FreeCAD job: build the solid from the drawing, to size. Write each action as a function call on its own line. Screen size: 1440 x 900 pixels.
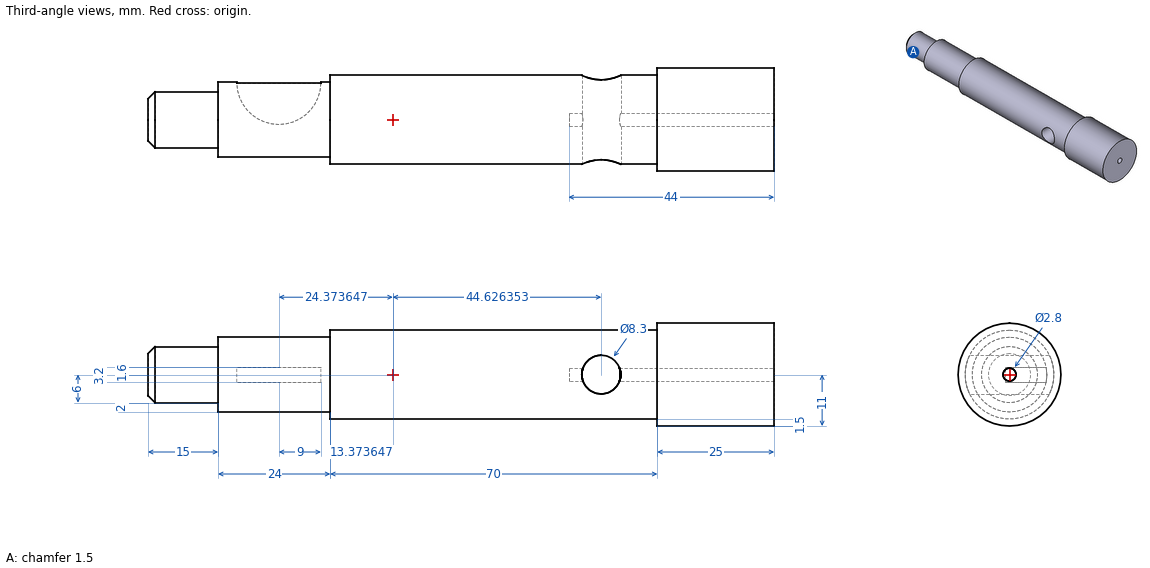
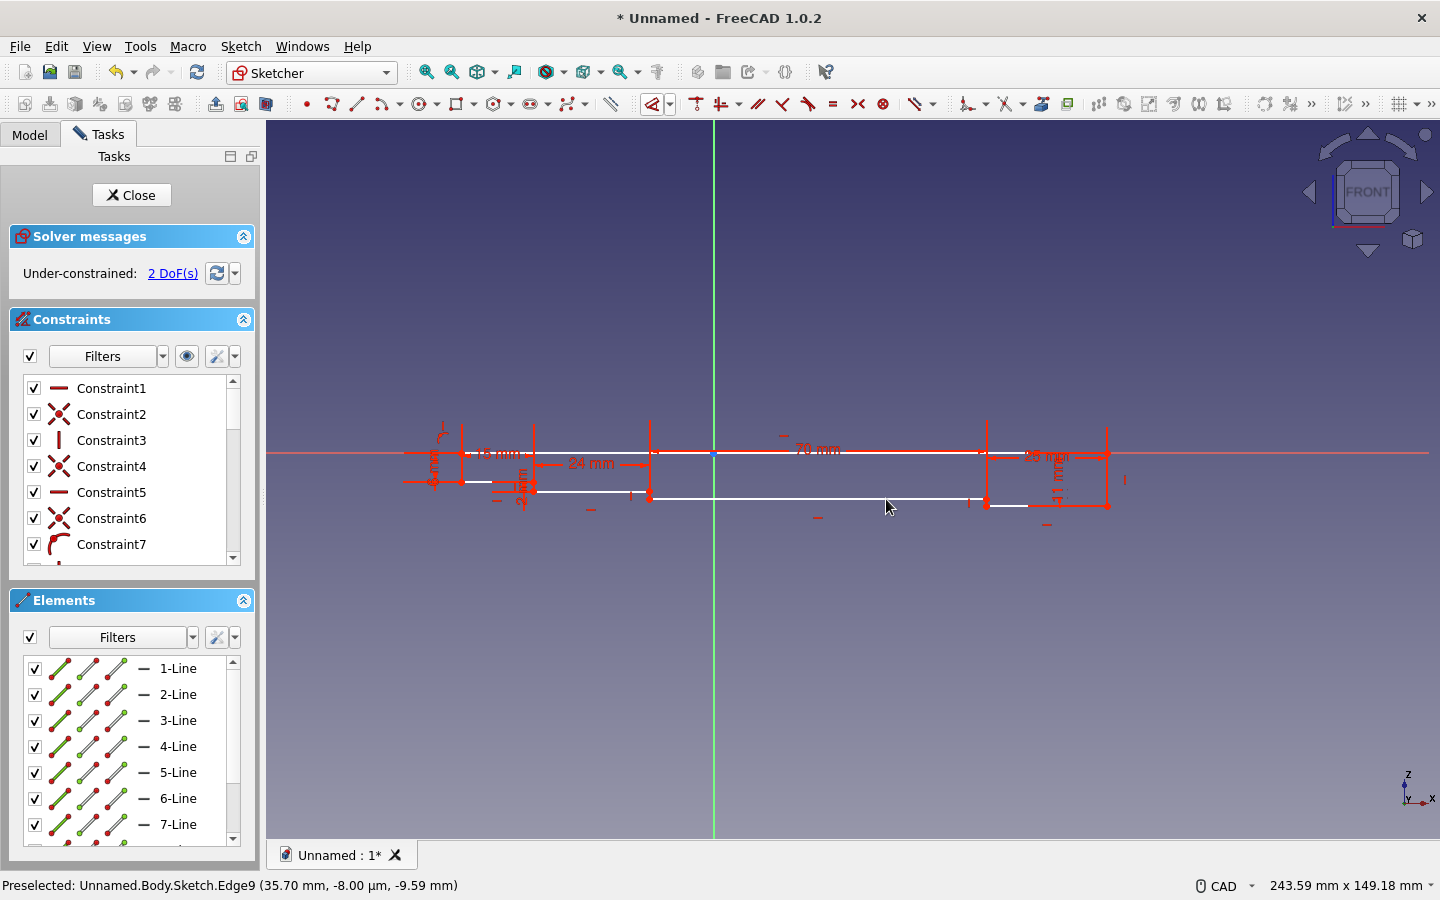
scroll(987, 503, up, 9)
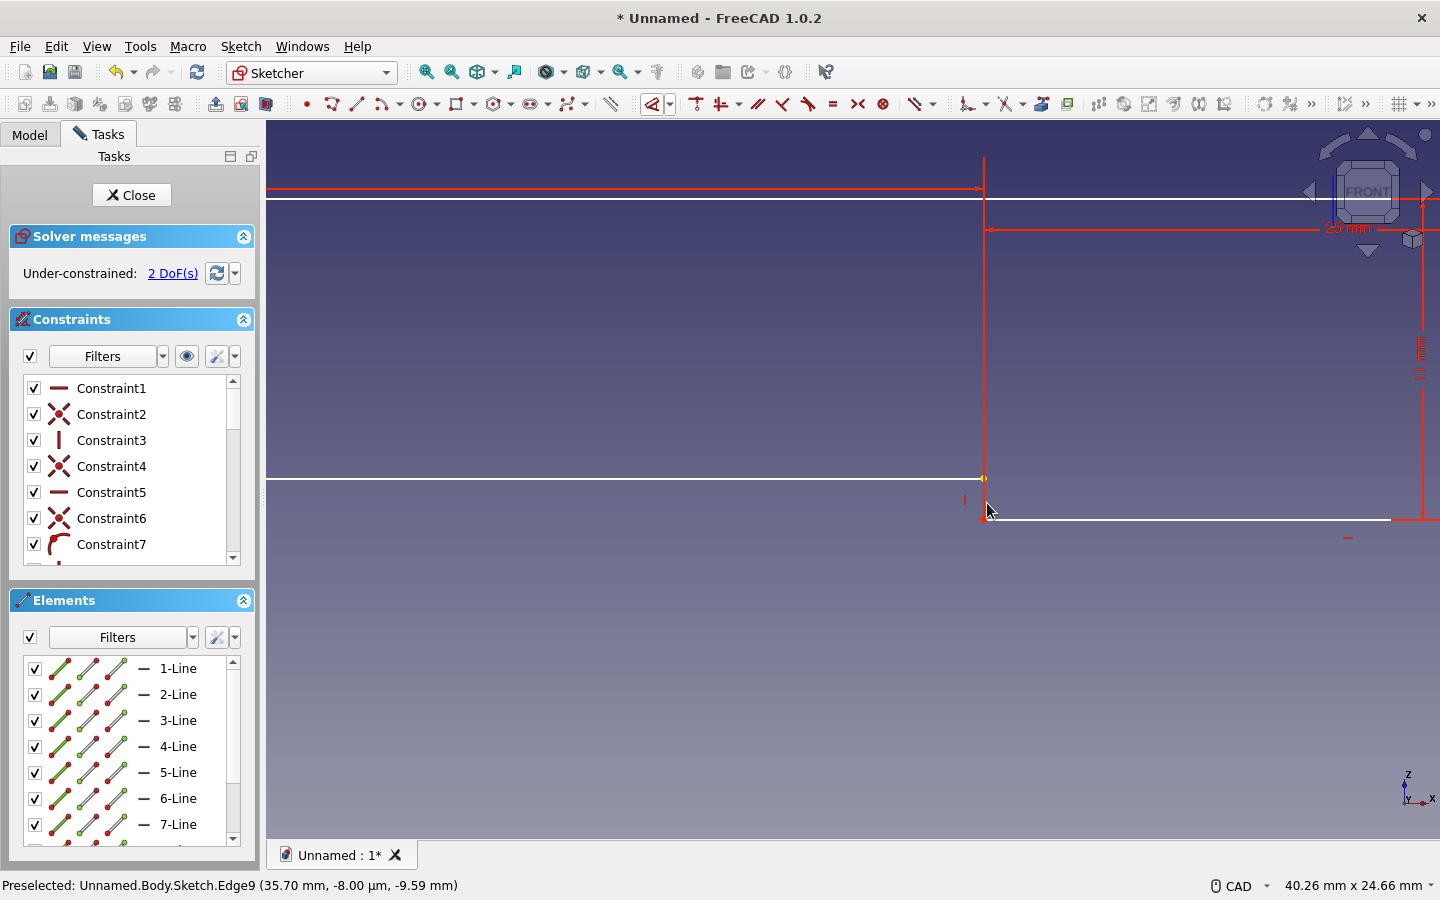
click(984, 499)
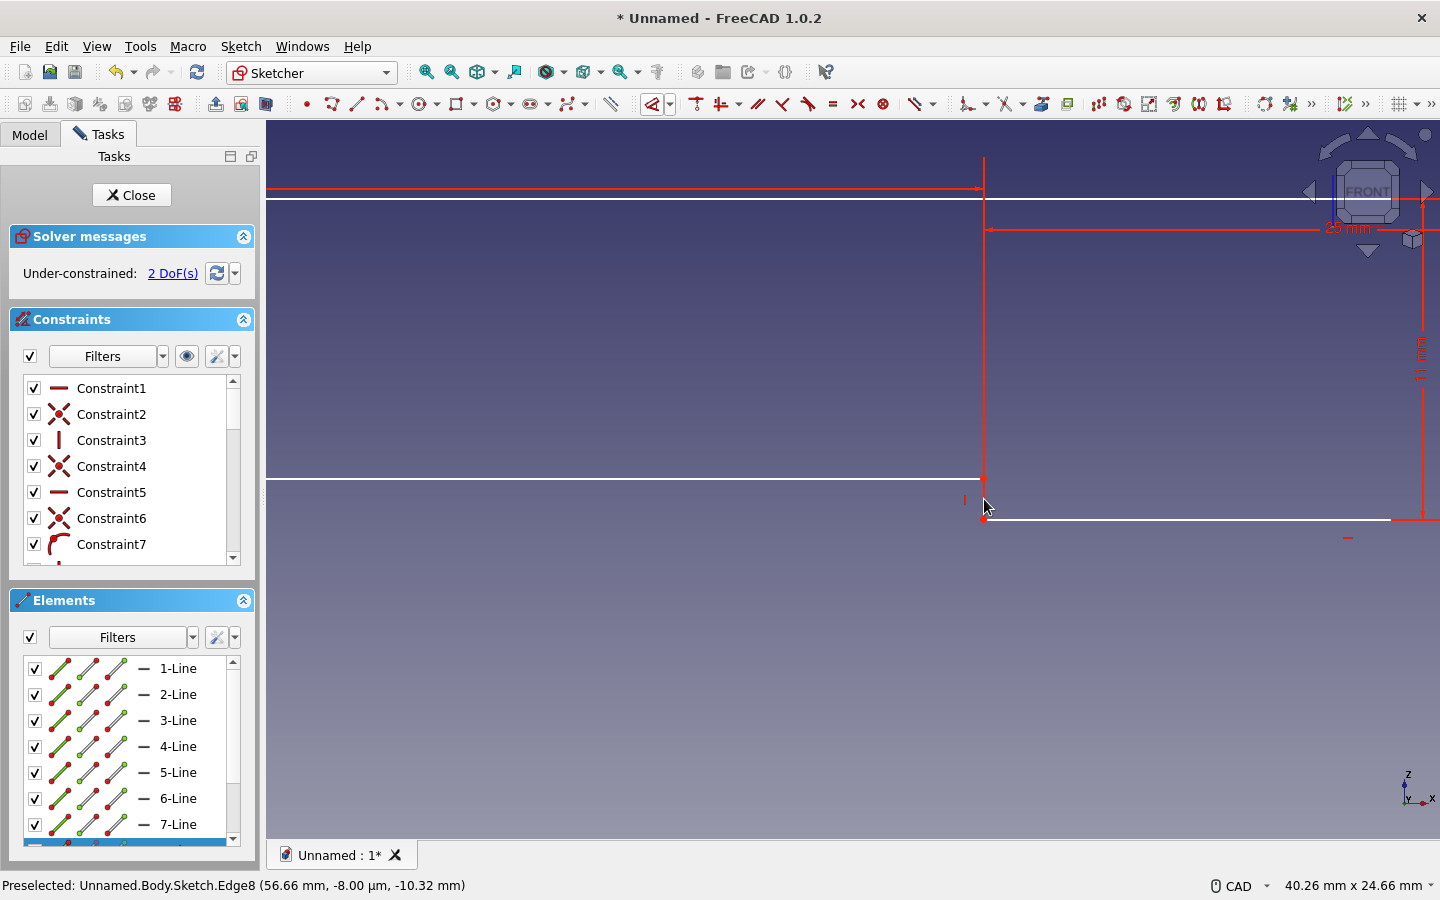
click(670, 104)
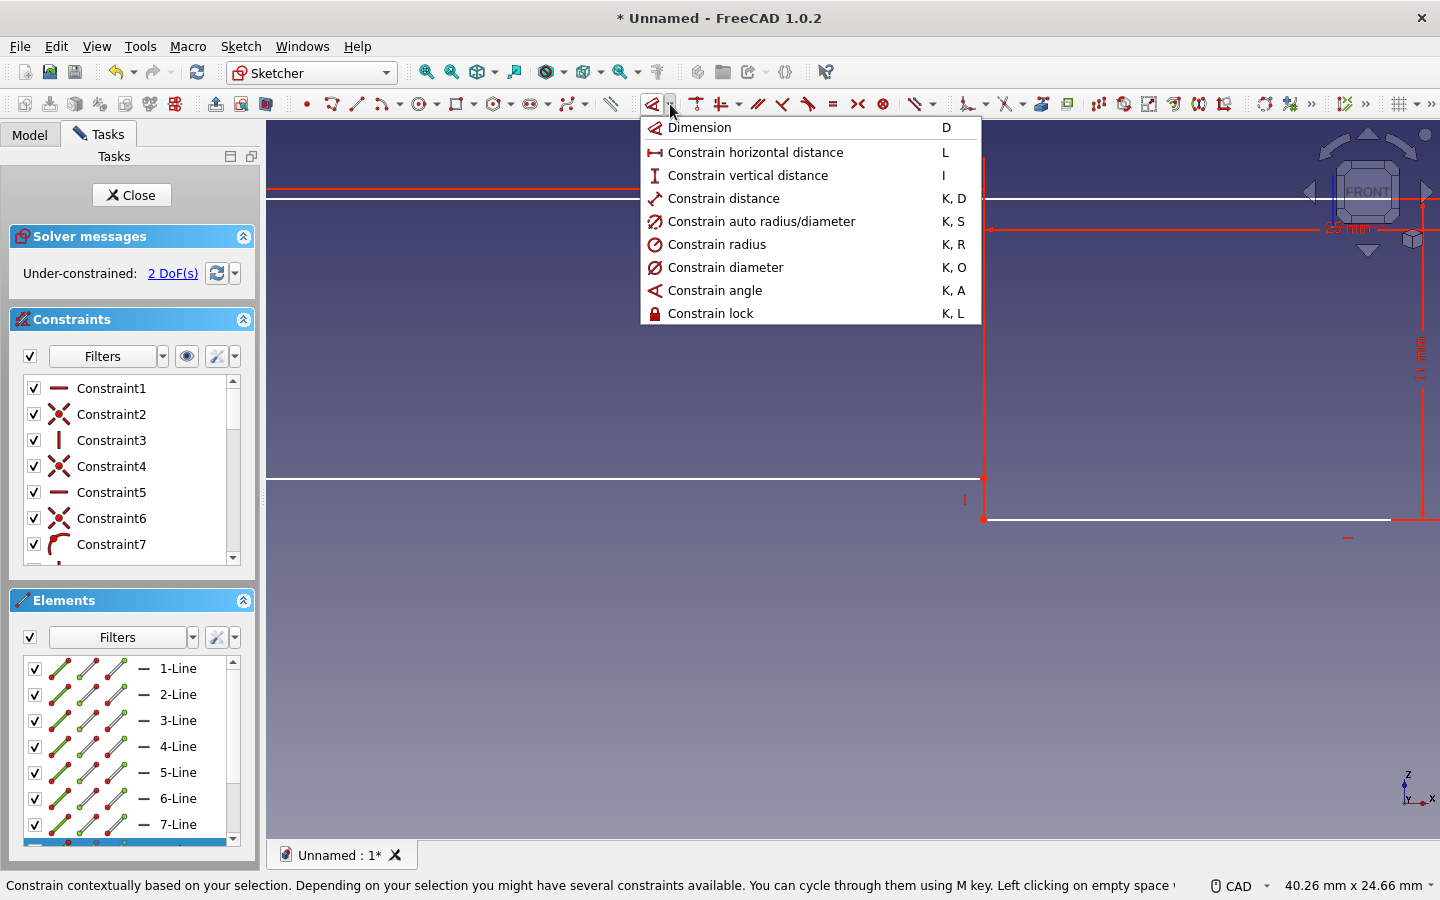
click(811, 176)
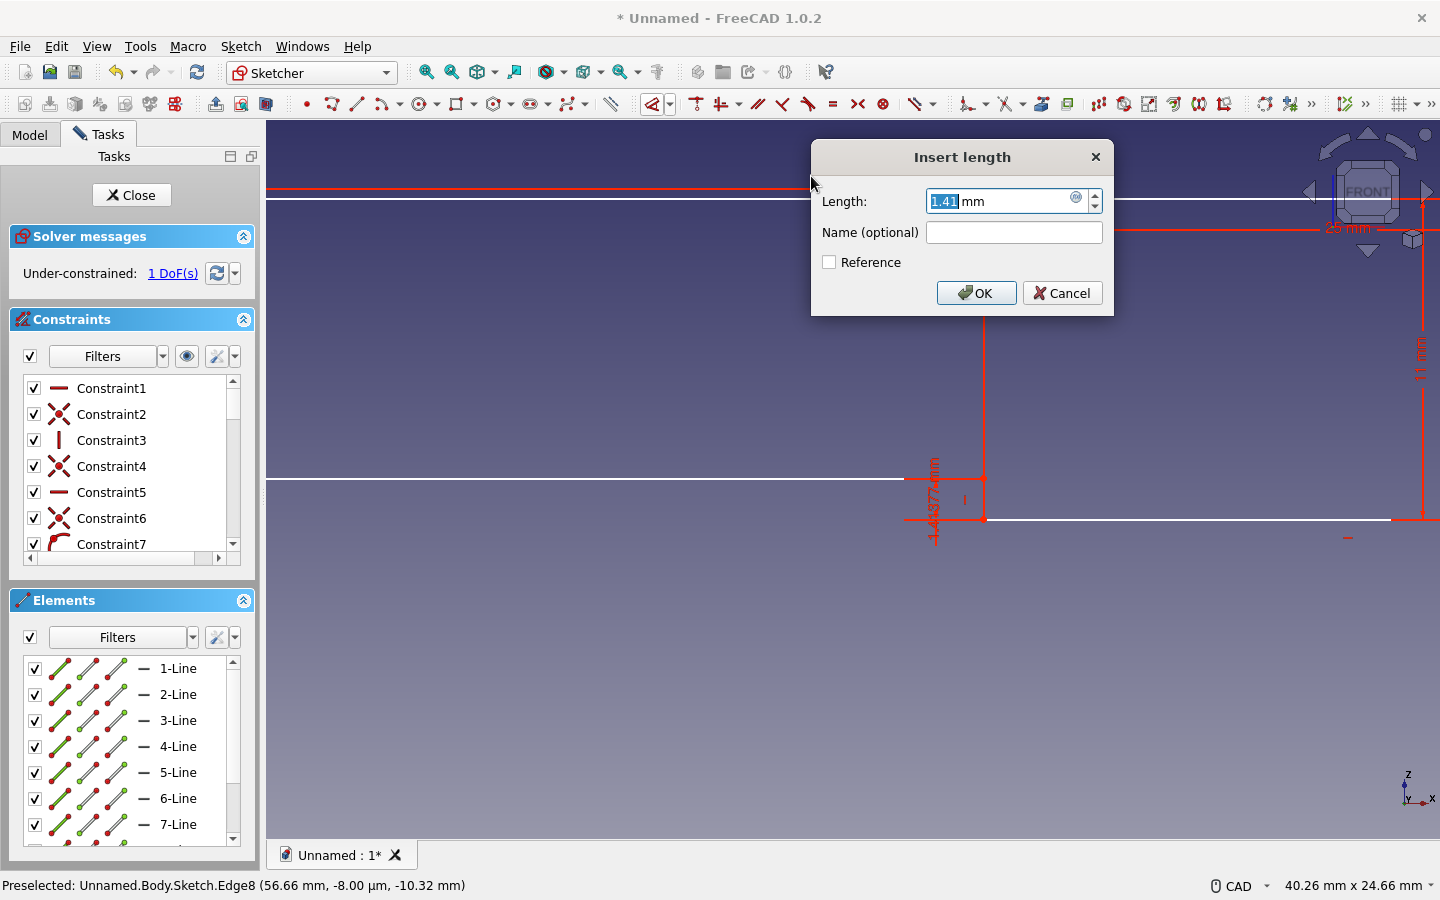
text(1.5)
key(Return)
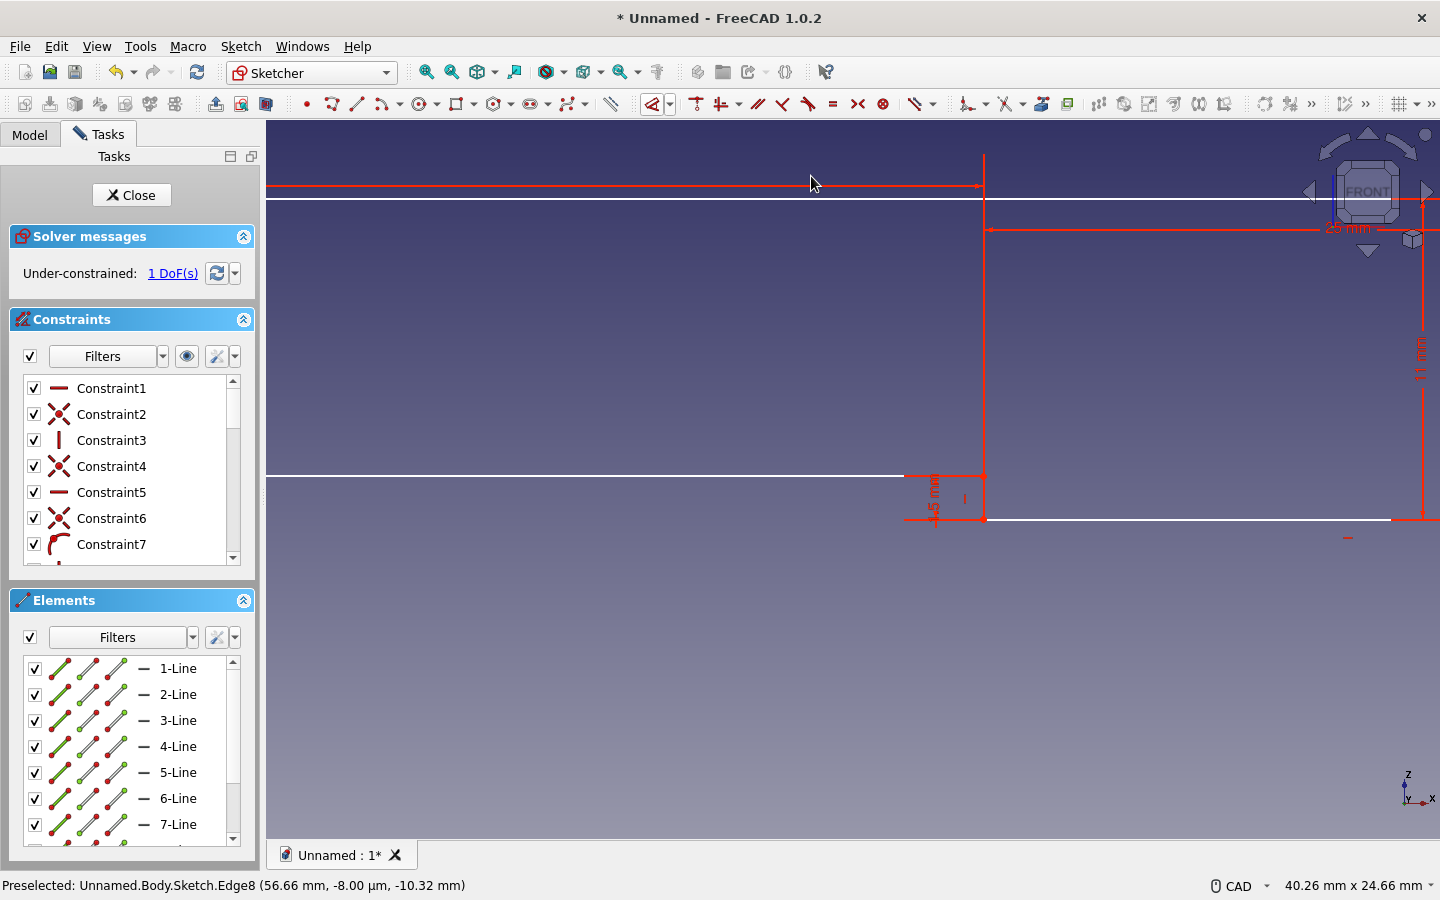
scroll(988, 503, down, 9)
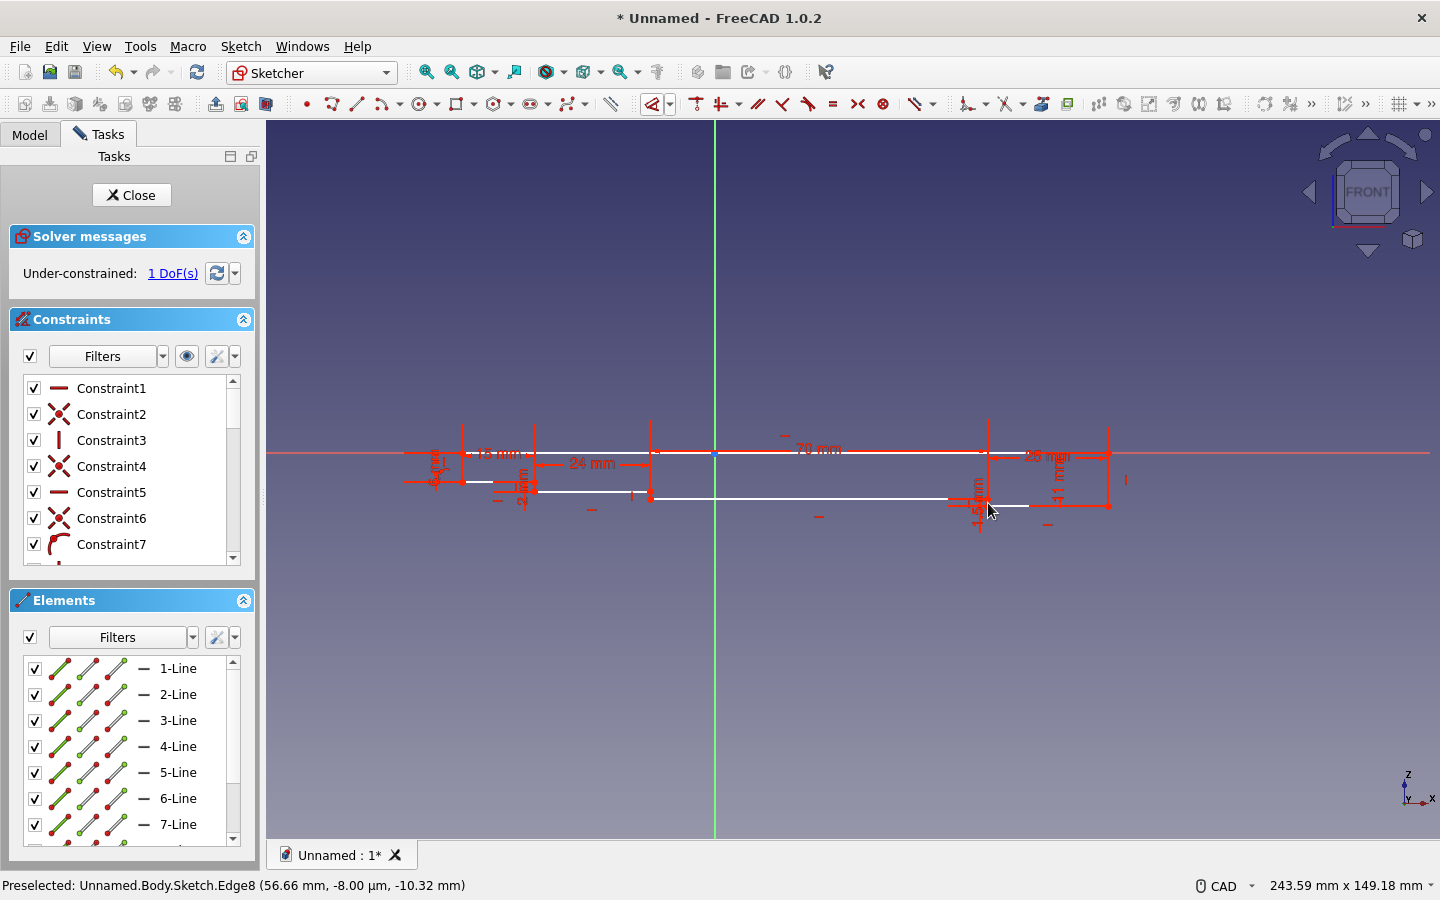
scroll(650, 492, up, 3)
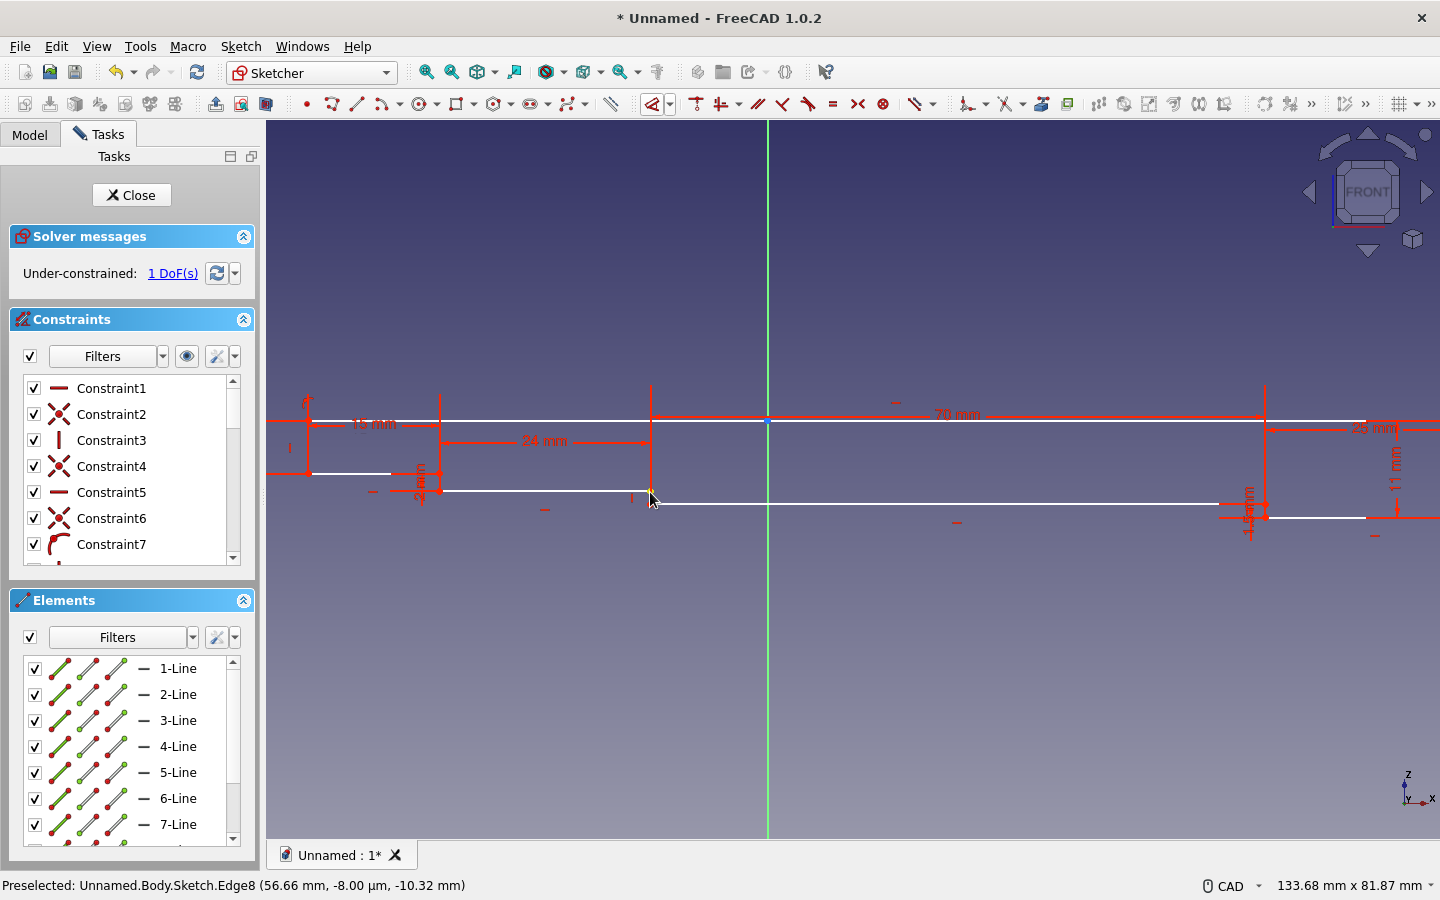
click(651, 491)